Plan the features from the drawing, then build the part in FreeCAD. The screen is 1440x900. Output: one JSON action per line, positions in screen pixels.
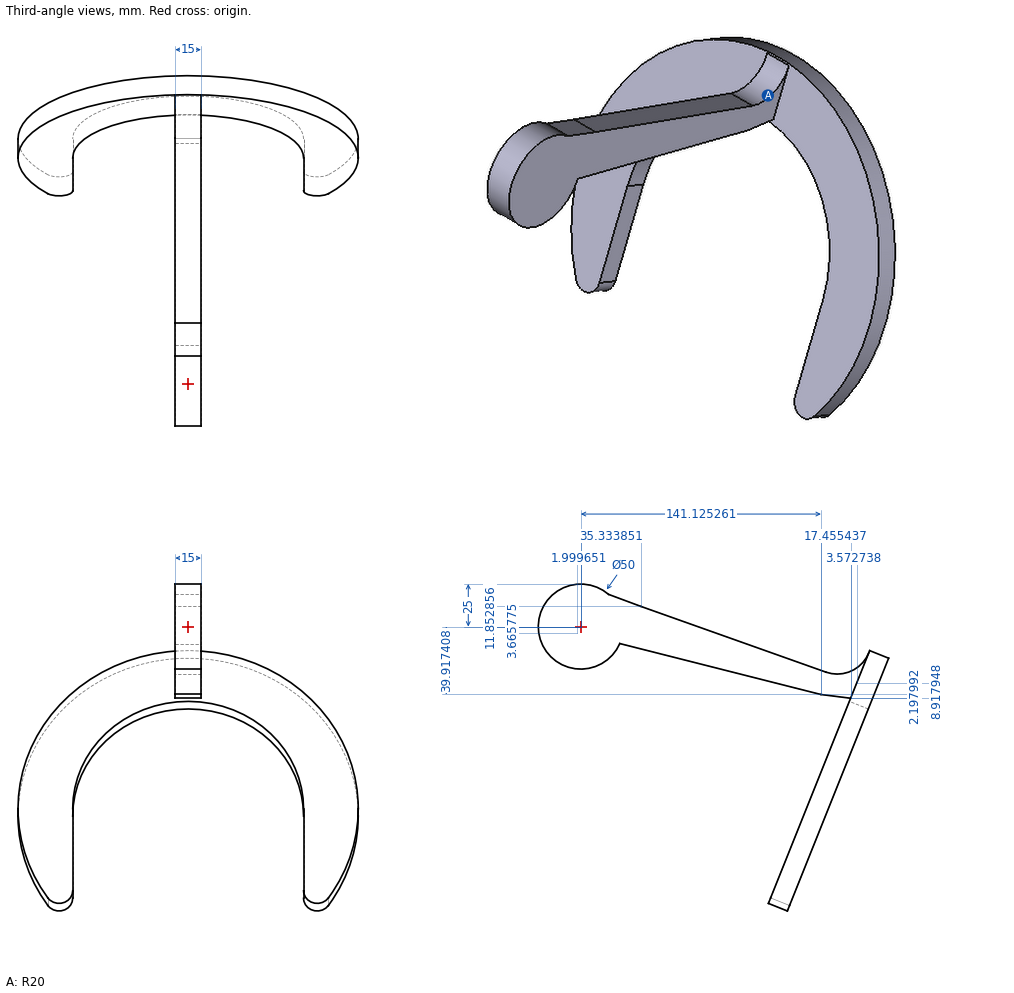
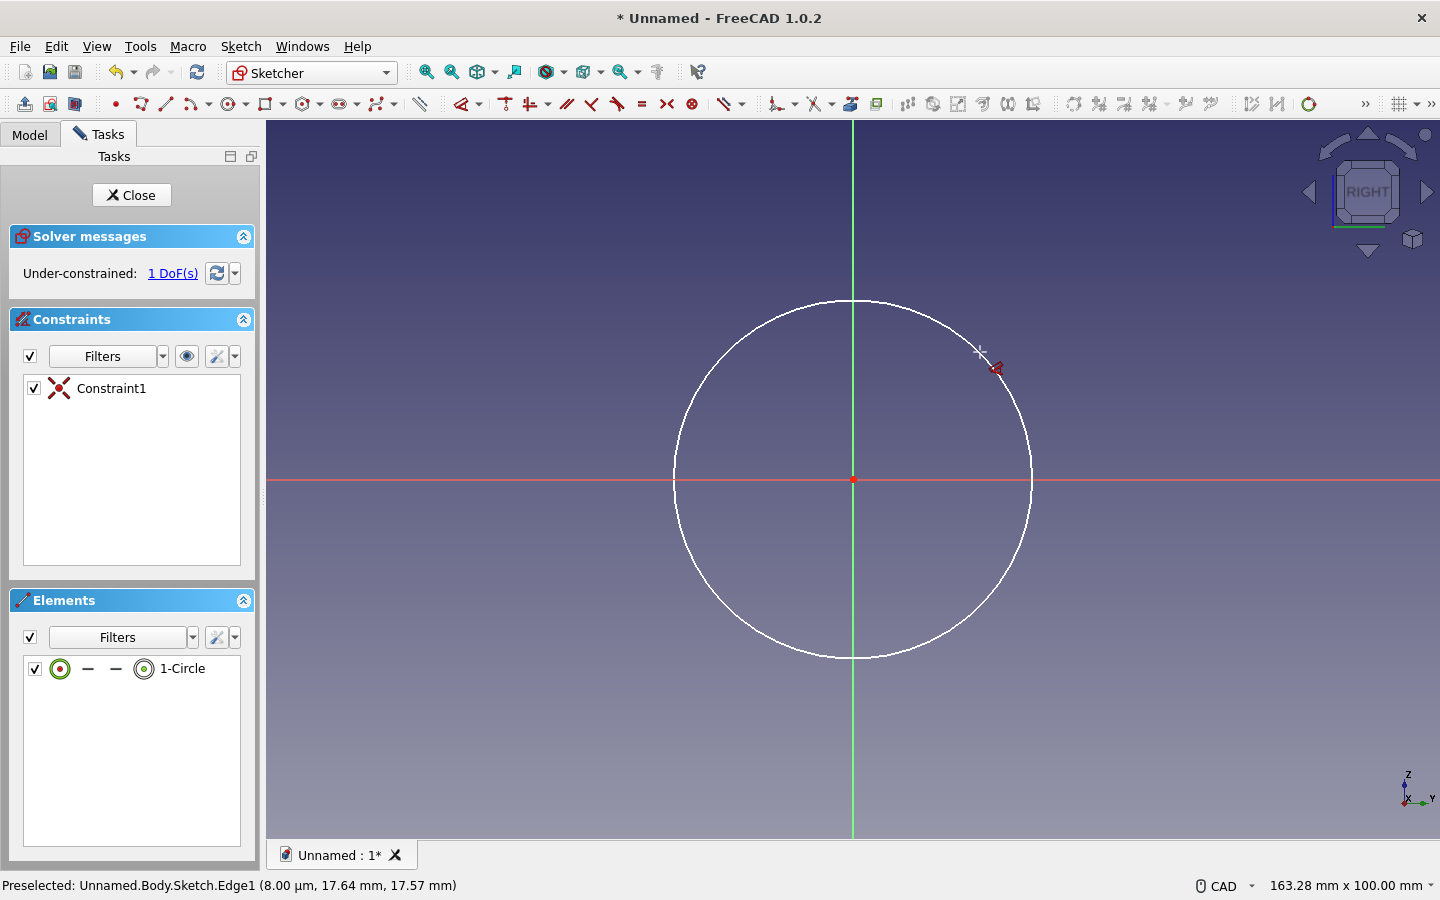
{"action": "left_click", "coordinate": [979, 352]}
{"action": "left_click", "coordinate": [1001, 329]}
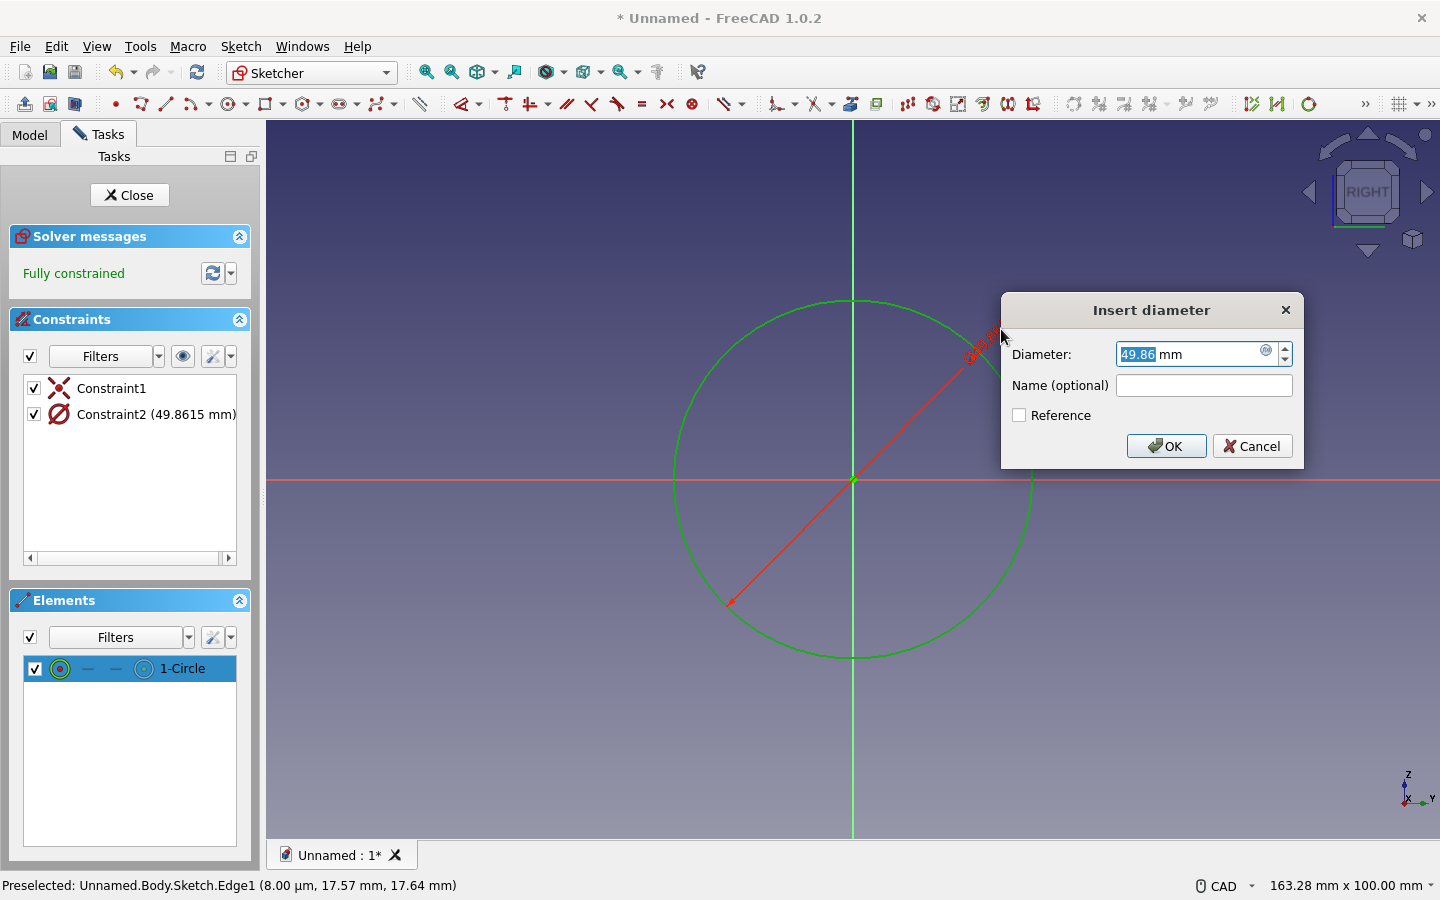
{"action": "type", "text": "50"}
{"action": "key", "text": "Return"}
{"action": "key", "text": "Escape"}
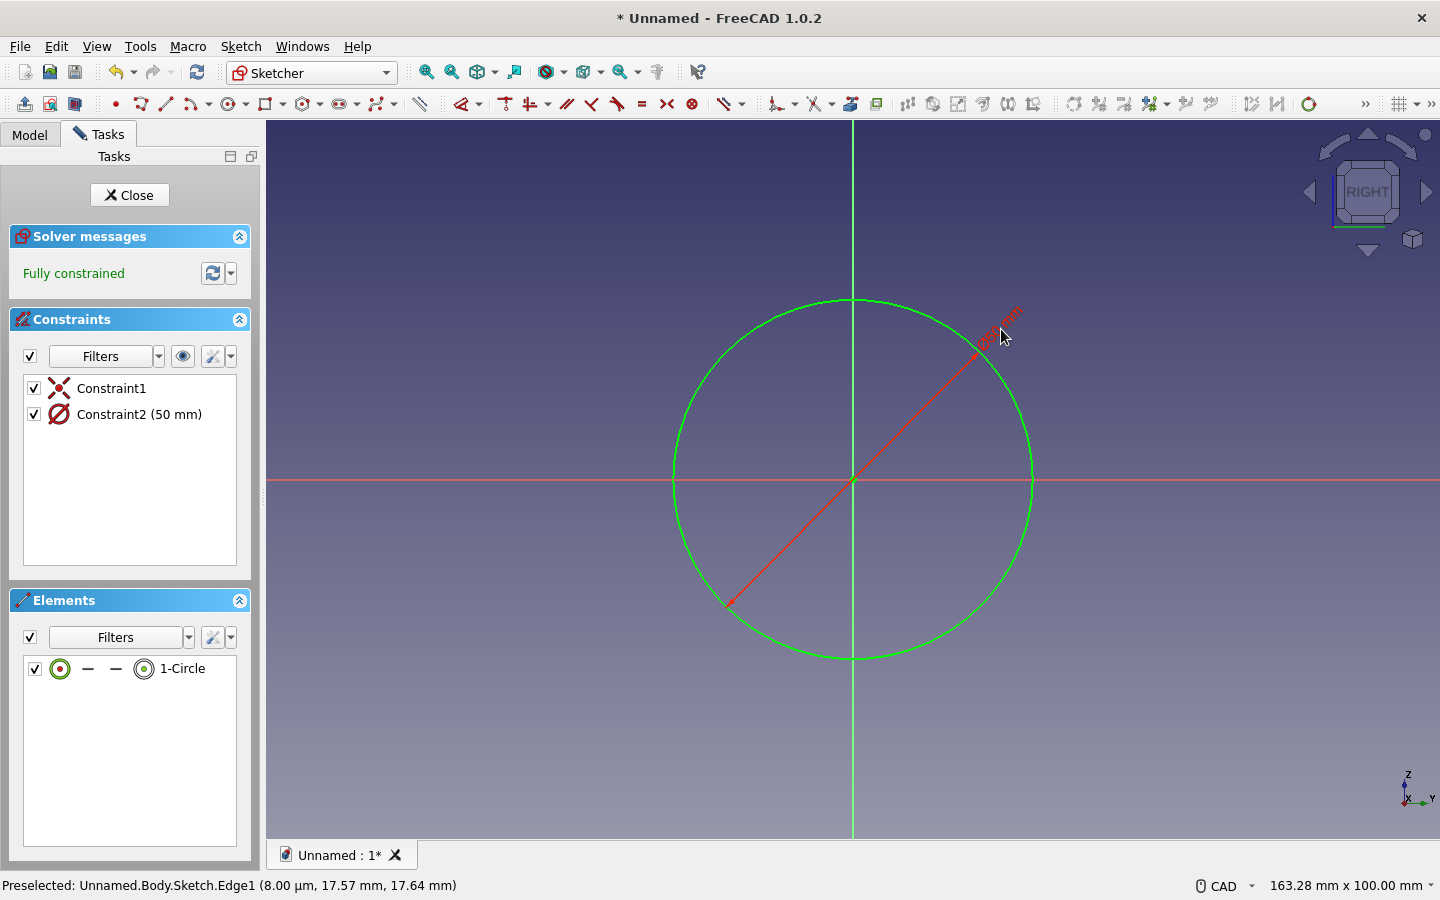
{"action": "left_click", "coordinate": [130, 195]}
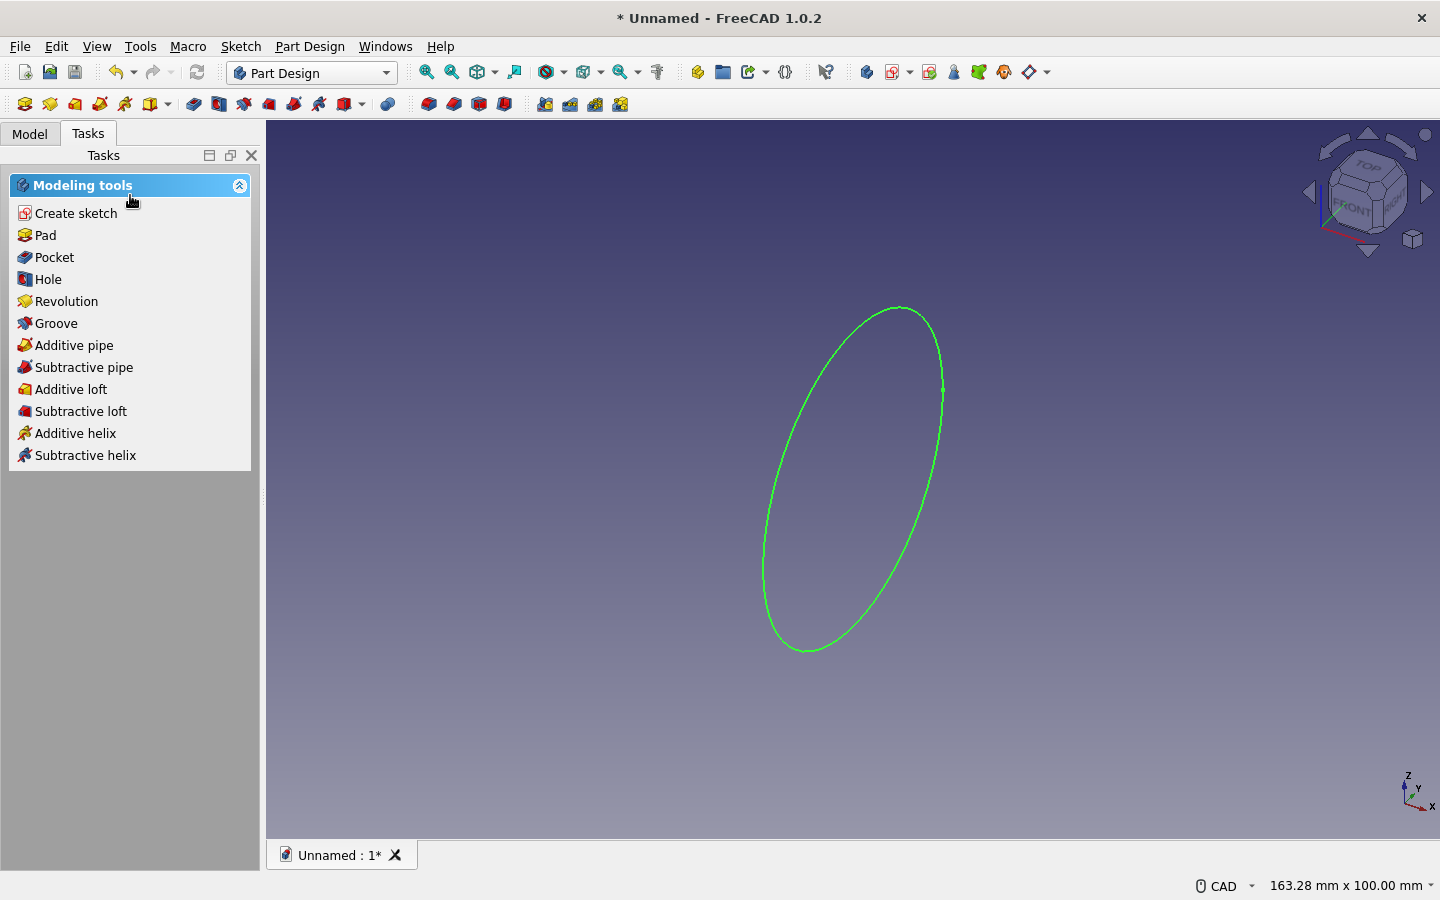
{"action": "left_click", "coordinate": [25, 104]}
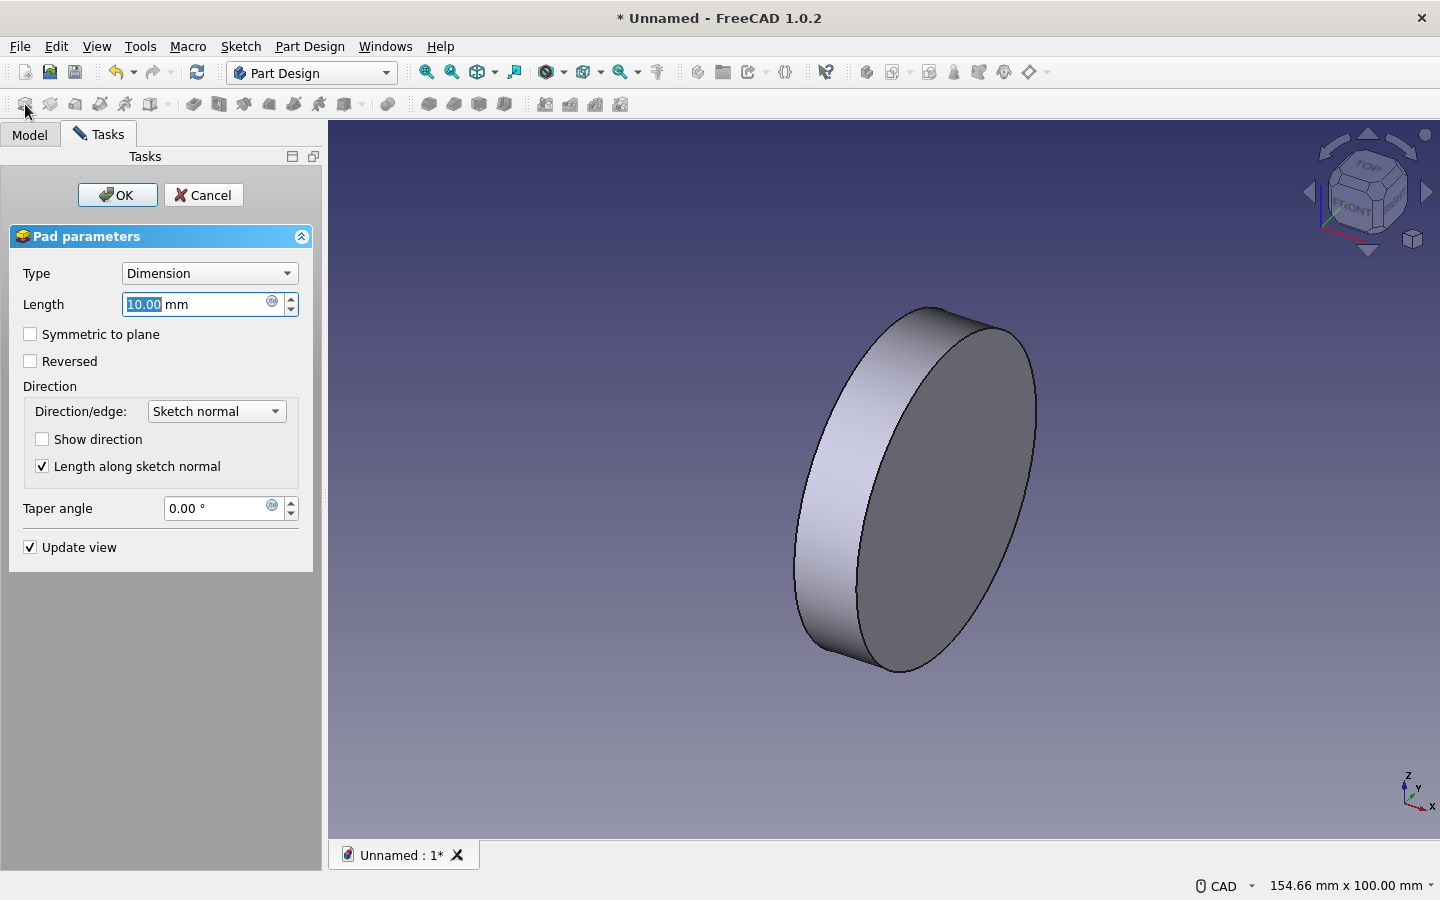
{"action": "type", "text": "15"}
{"action": "key", "text": "Tab"}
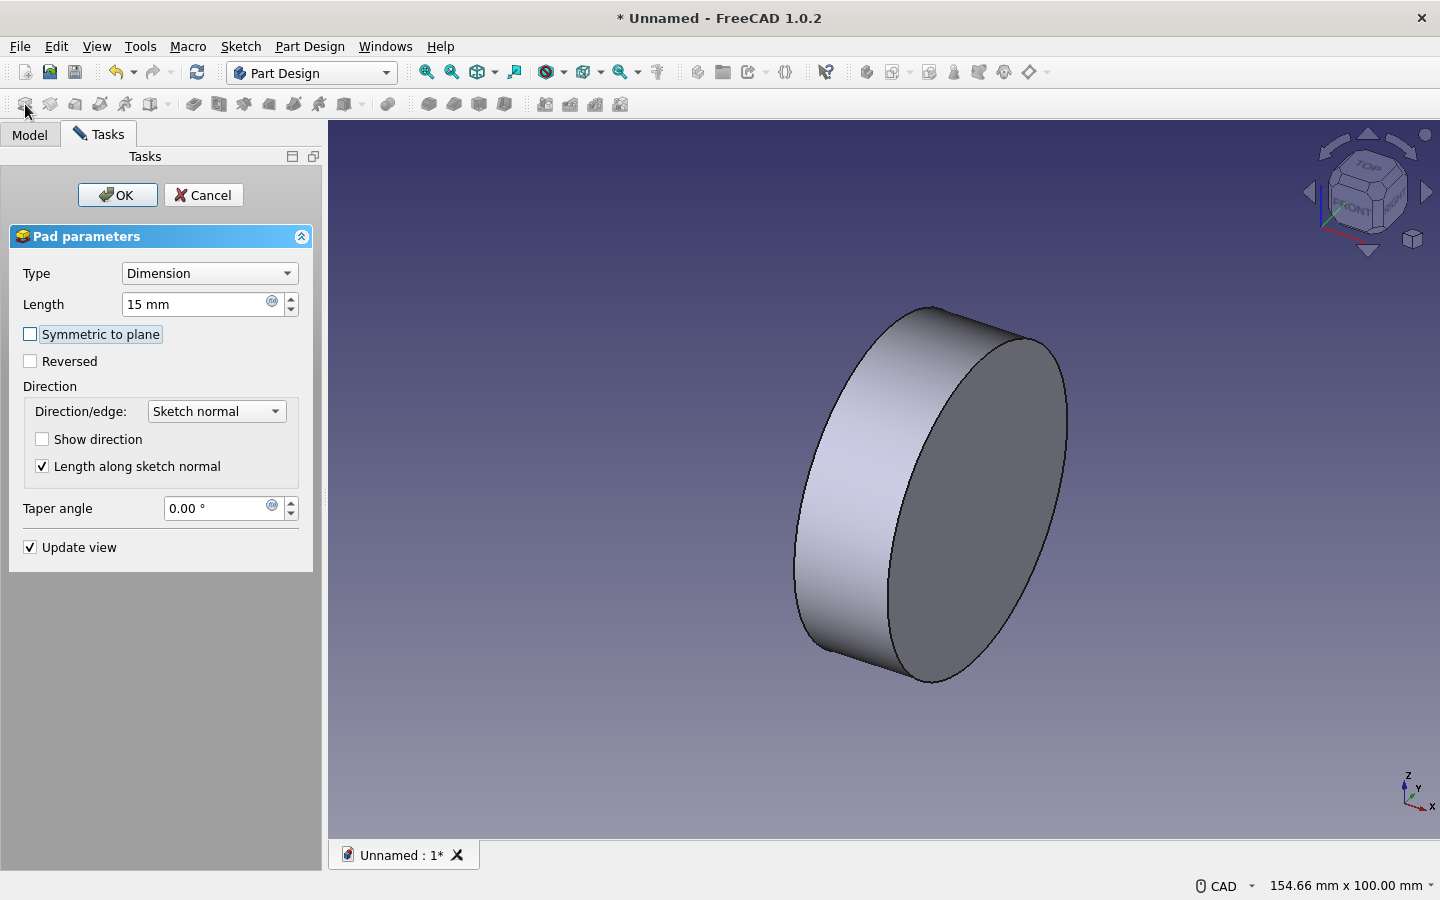
{"action": "left_click", "coordinate": [31, 334]}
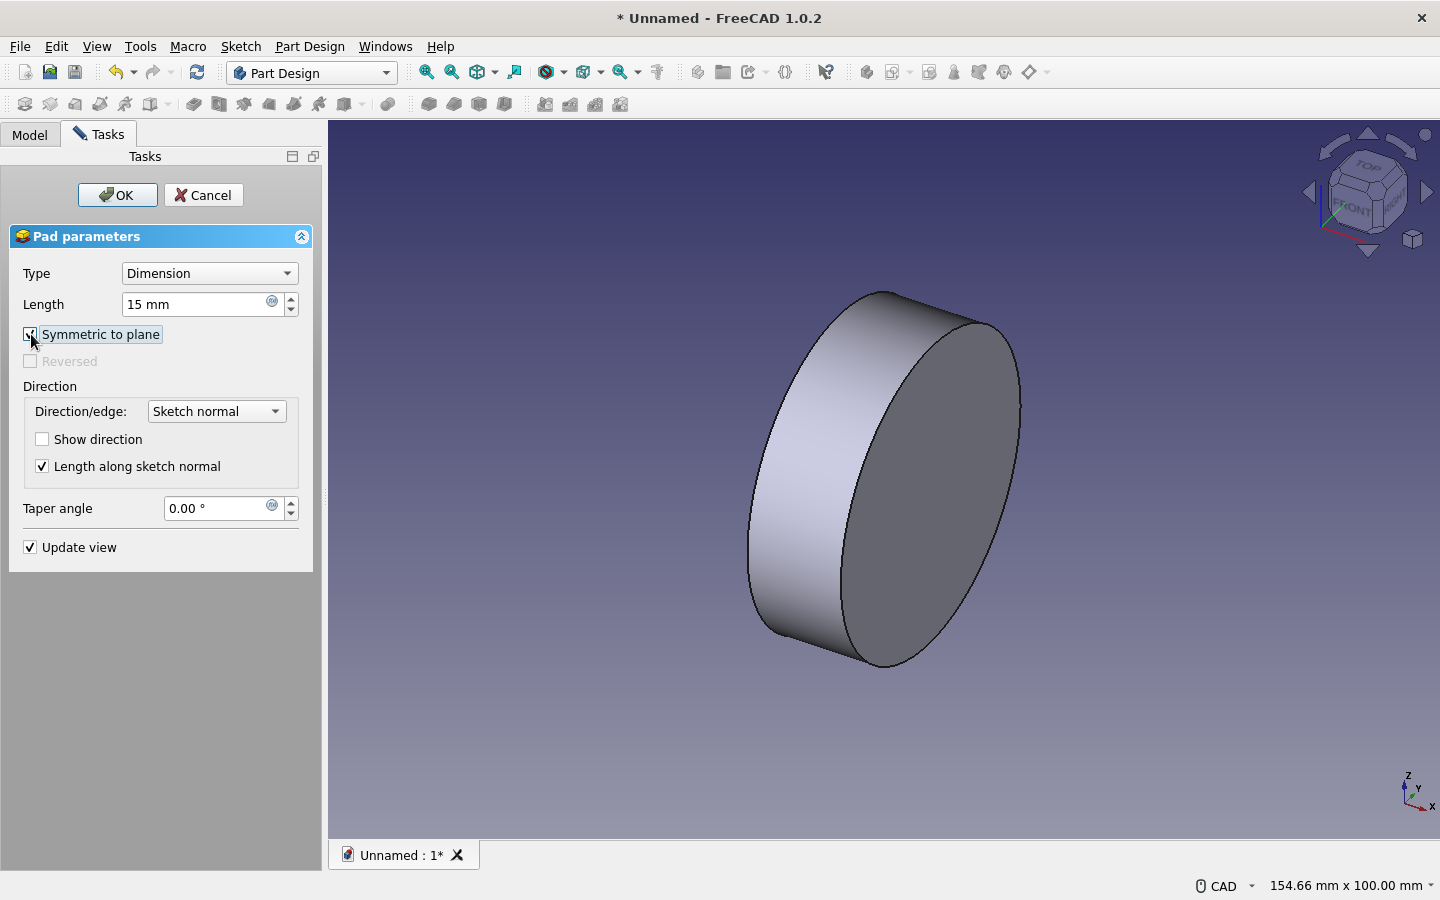
{"action": "left_click", "coordinate": [118, 195]}